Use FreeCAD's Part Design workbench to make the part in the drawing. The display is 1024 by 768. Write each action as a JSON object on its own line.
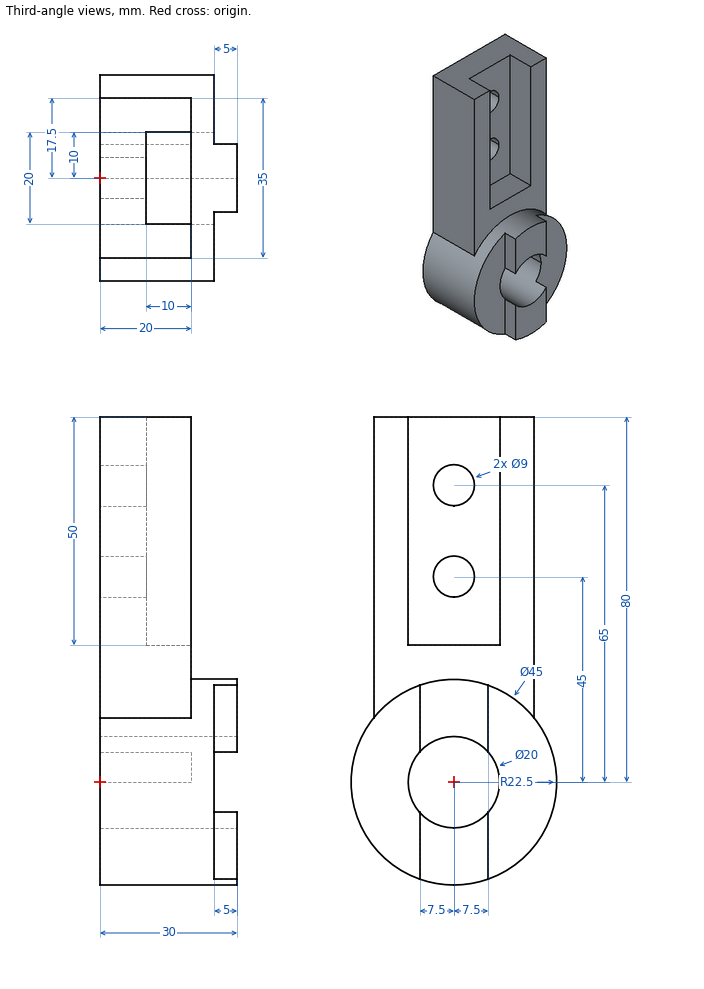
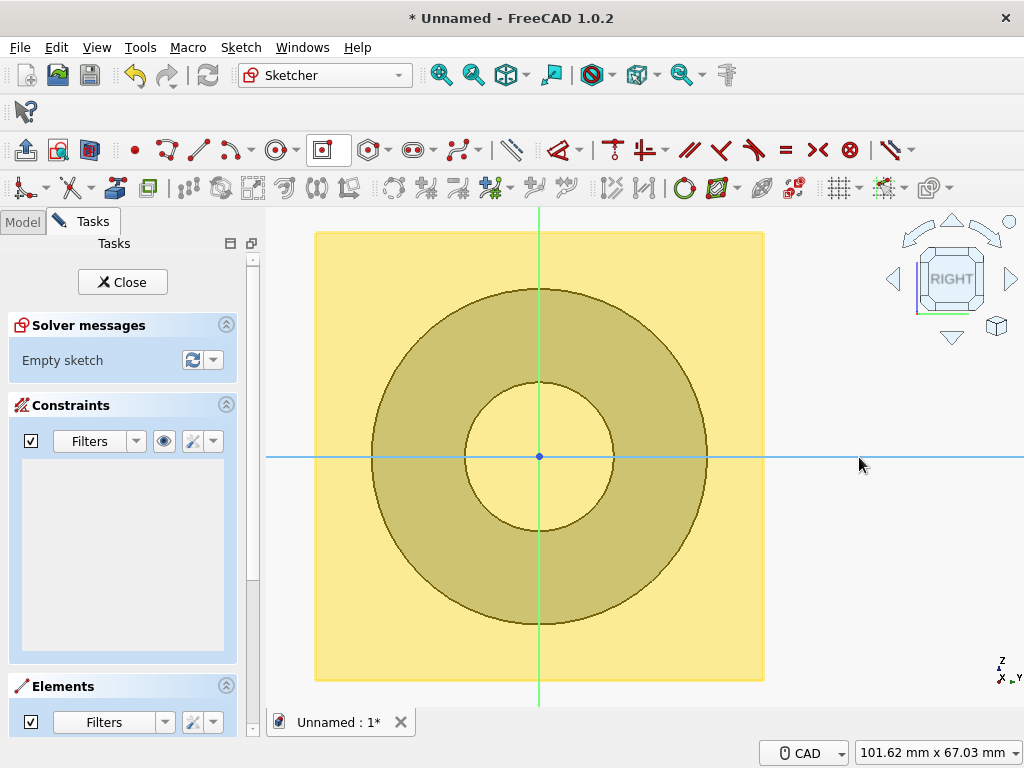
{"action": "left_click", "coordinate": [200, 150]}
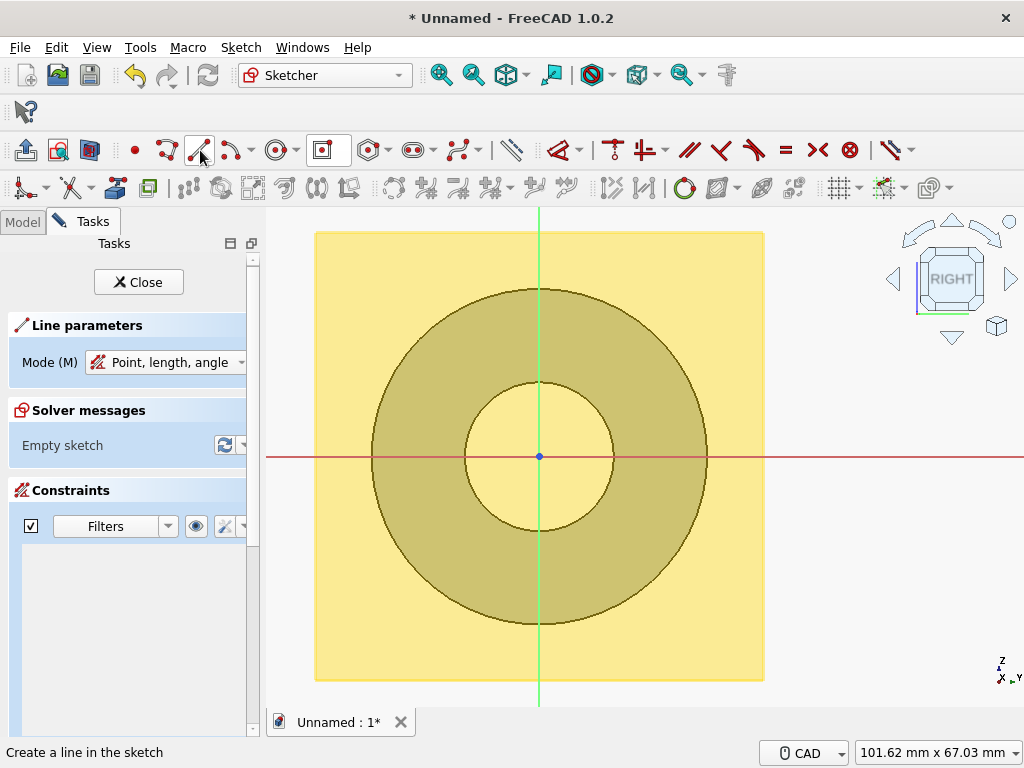
{"action": "left_click", "coordinate": [595, 299]}
{"action": "left_click", "coordinate": [595, 615]}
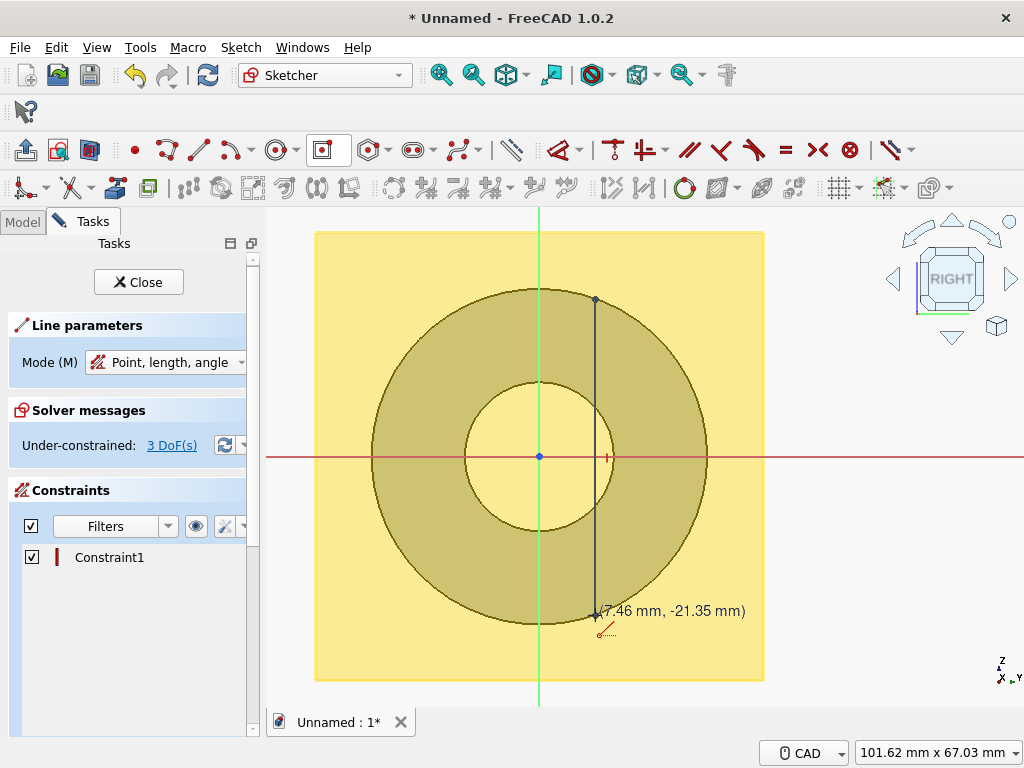
{"action": "left_click", "coordinate": [254, 150]}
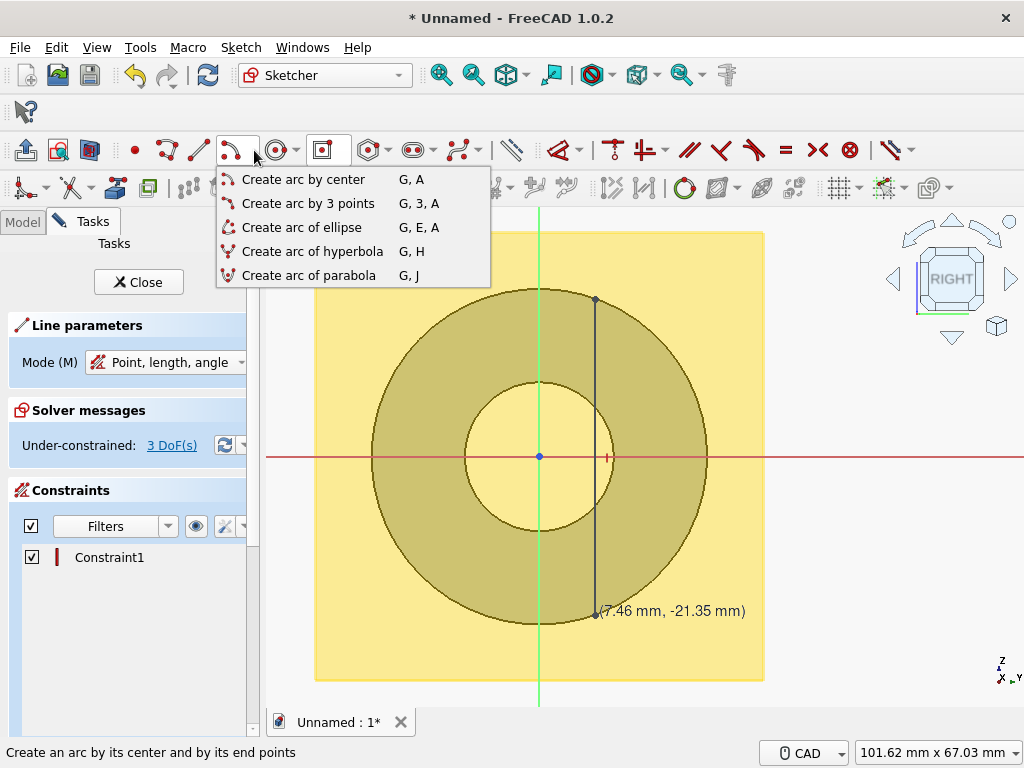
{"action": "left_click", "coordinate": [354, 203]}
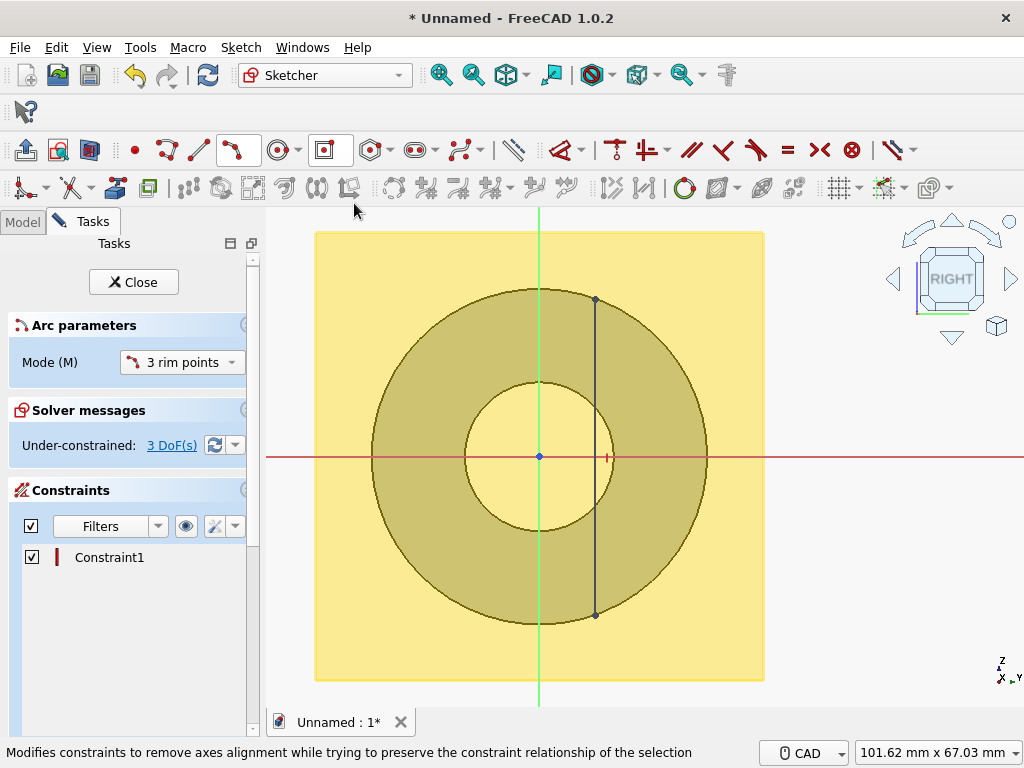
{"action": "left_click", "coordinate": [595, 616]}
{"action": "left_click", "coordinate": [595, 300]}
{"action": "left_click", "coordinate": [702, 498]}
{"action": "key", "text": "Escape"}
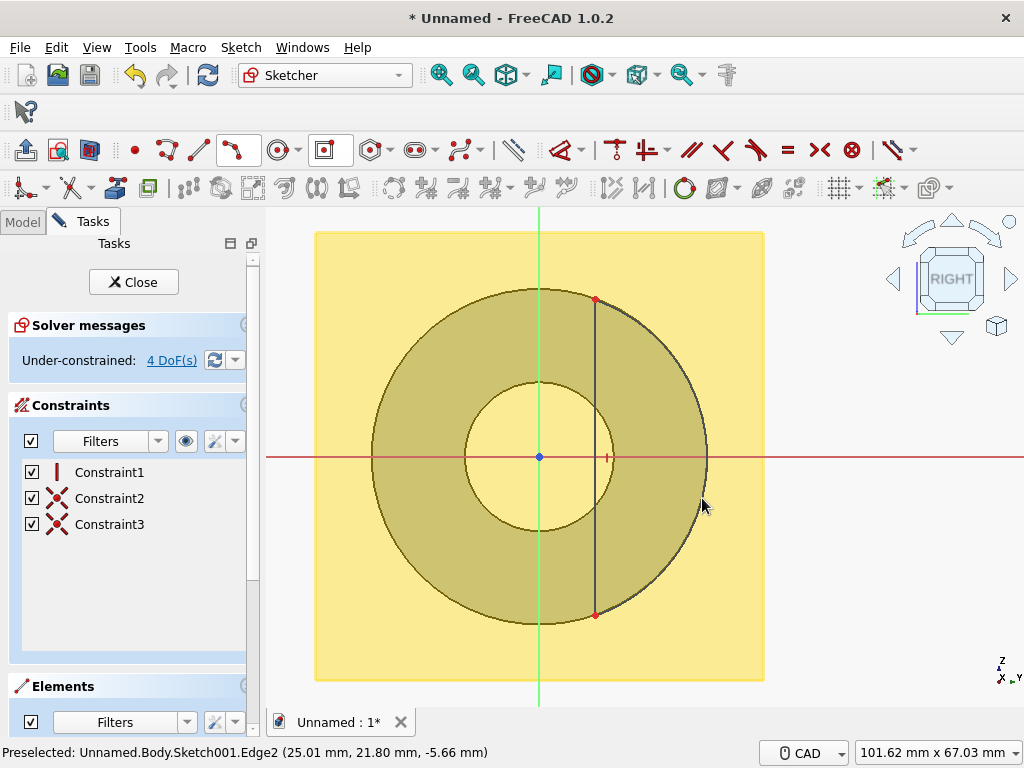
{"action": "left_click_drag", "start_coordinate": [529, 447], "coordinate": [550, 468]}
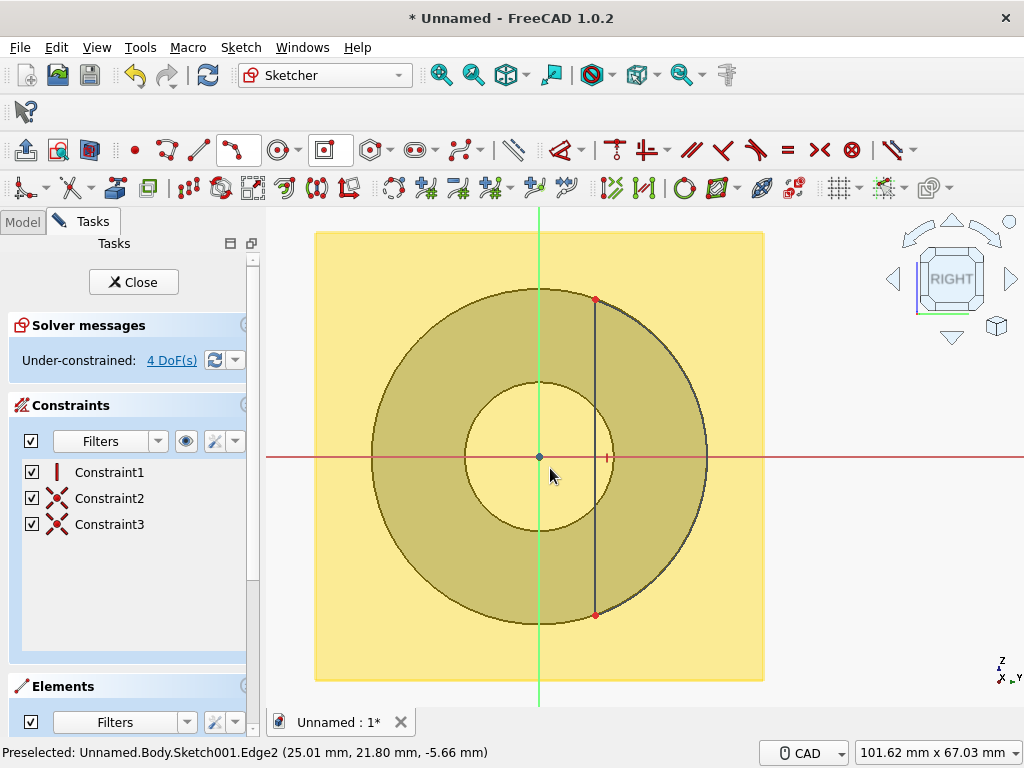
{"action": "left_click", "coordinate": [616, 150]}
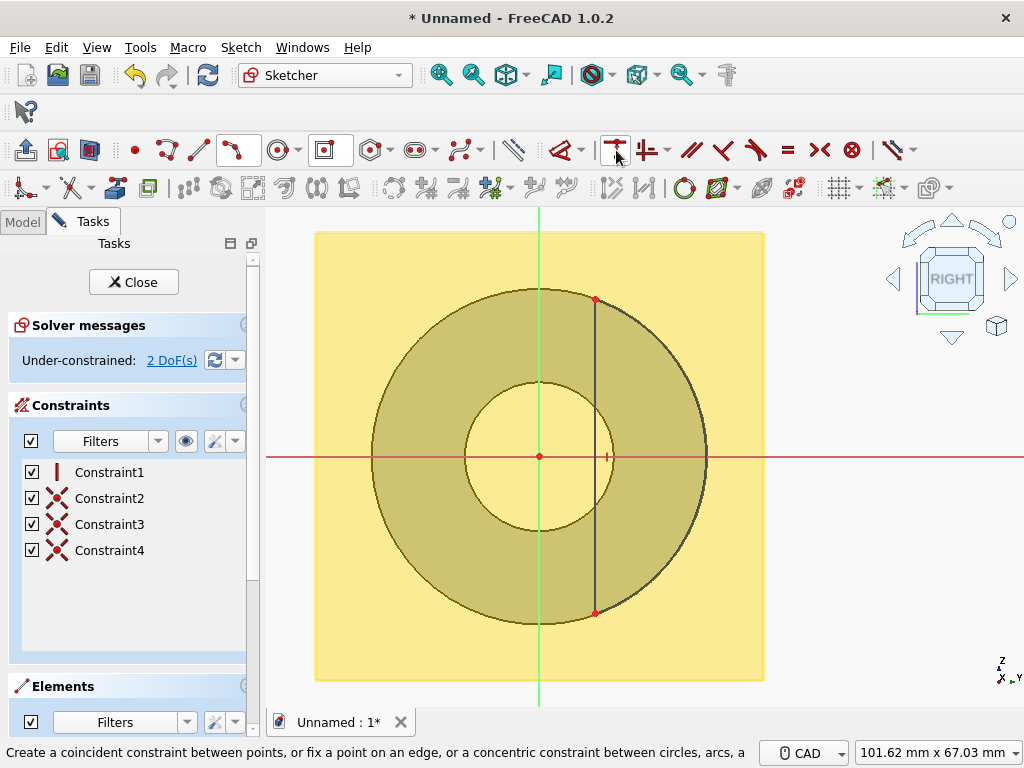
{"action": "left_click", "coordinate": [686, 536]}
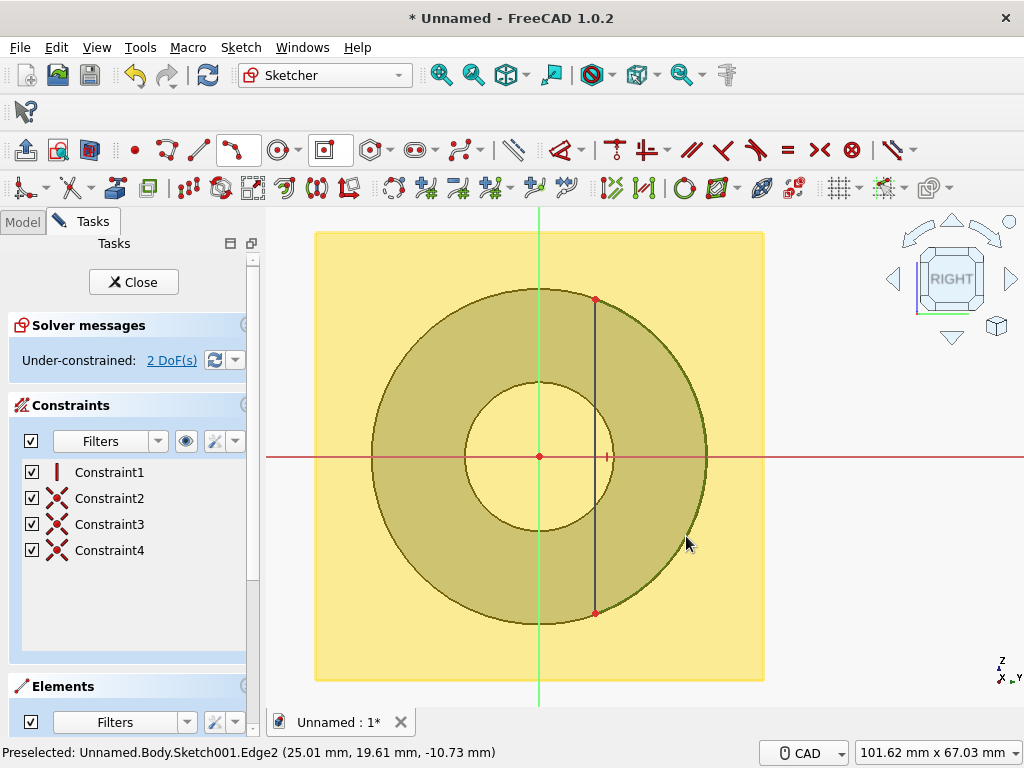
{"action": "left_click", "coordinate": [584, 150]}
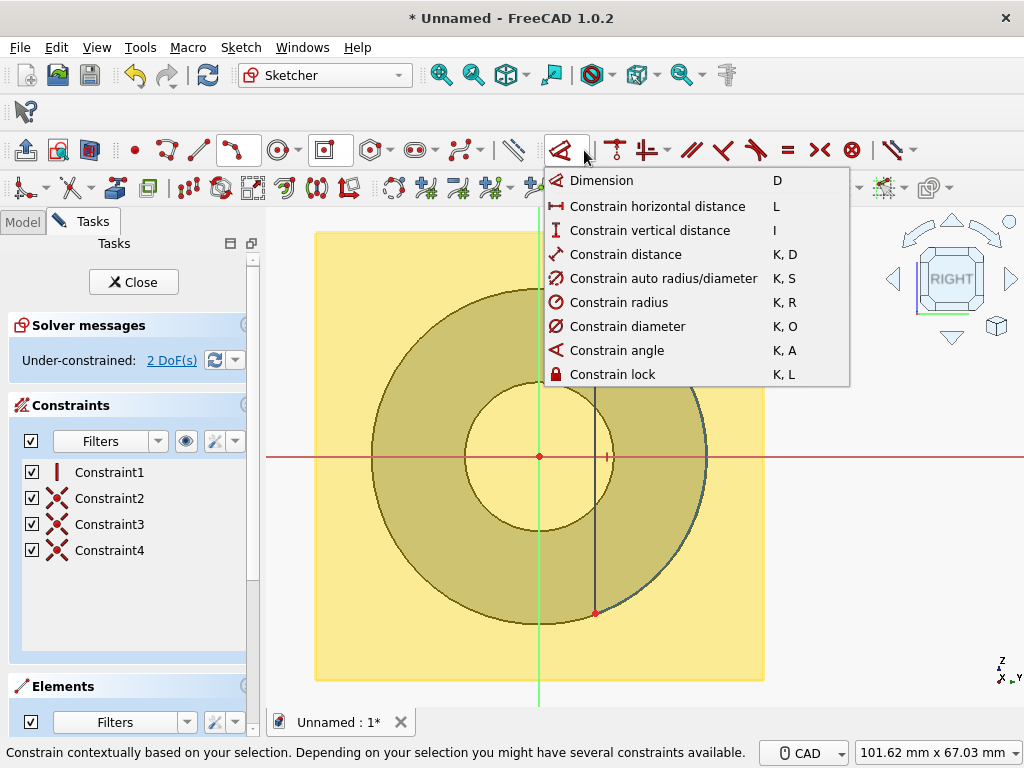
{"action": "left_click", "coordinate": [697, 302]}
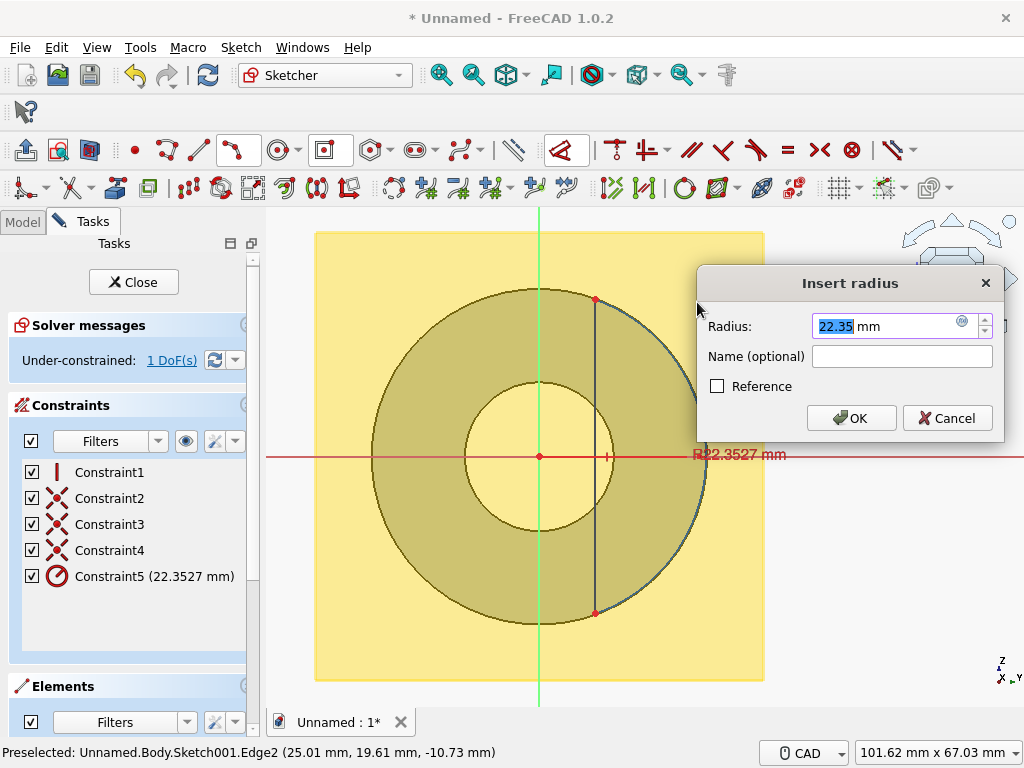
{"action": "type", "text": "22.5"}
{"action": "key", "text": "Return"}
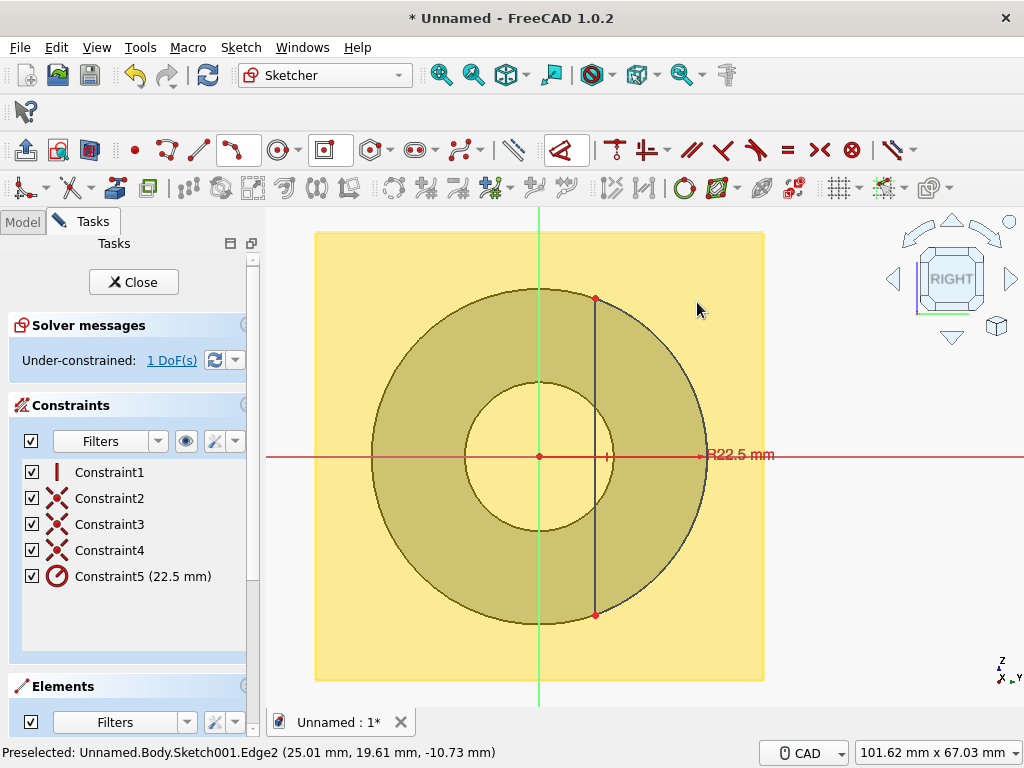
{"action": "left_click", "coordinate": [595, 298]}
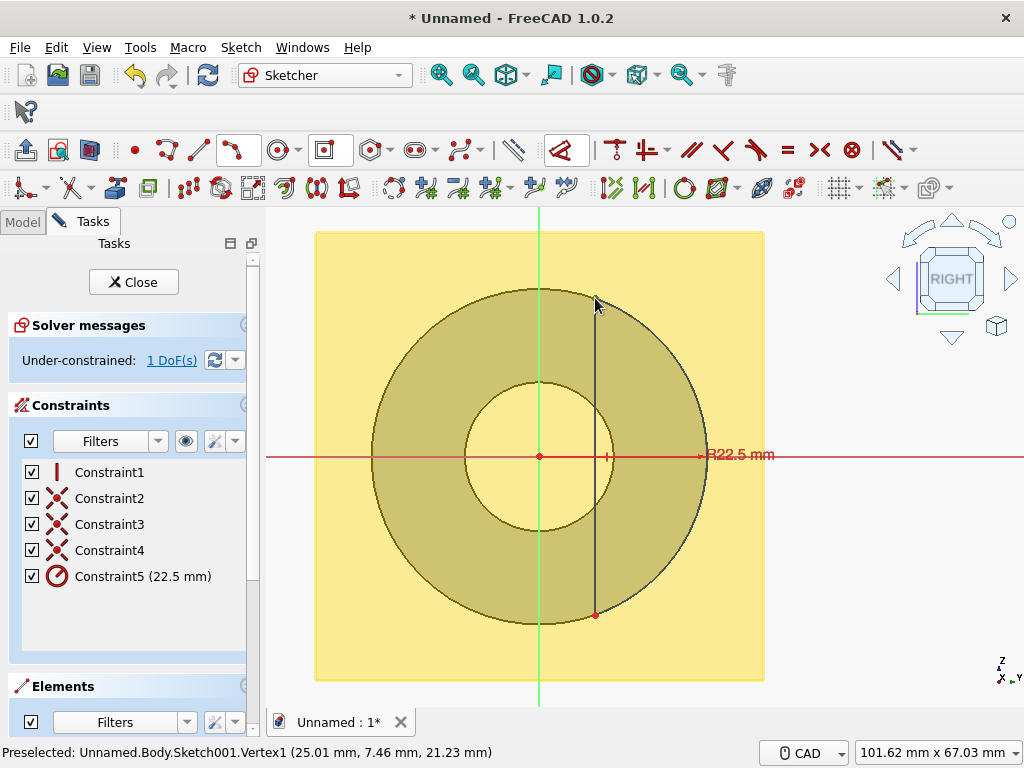
{"action": "key", "text": "l"}